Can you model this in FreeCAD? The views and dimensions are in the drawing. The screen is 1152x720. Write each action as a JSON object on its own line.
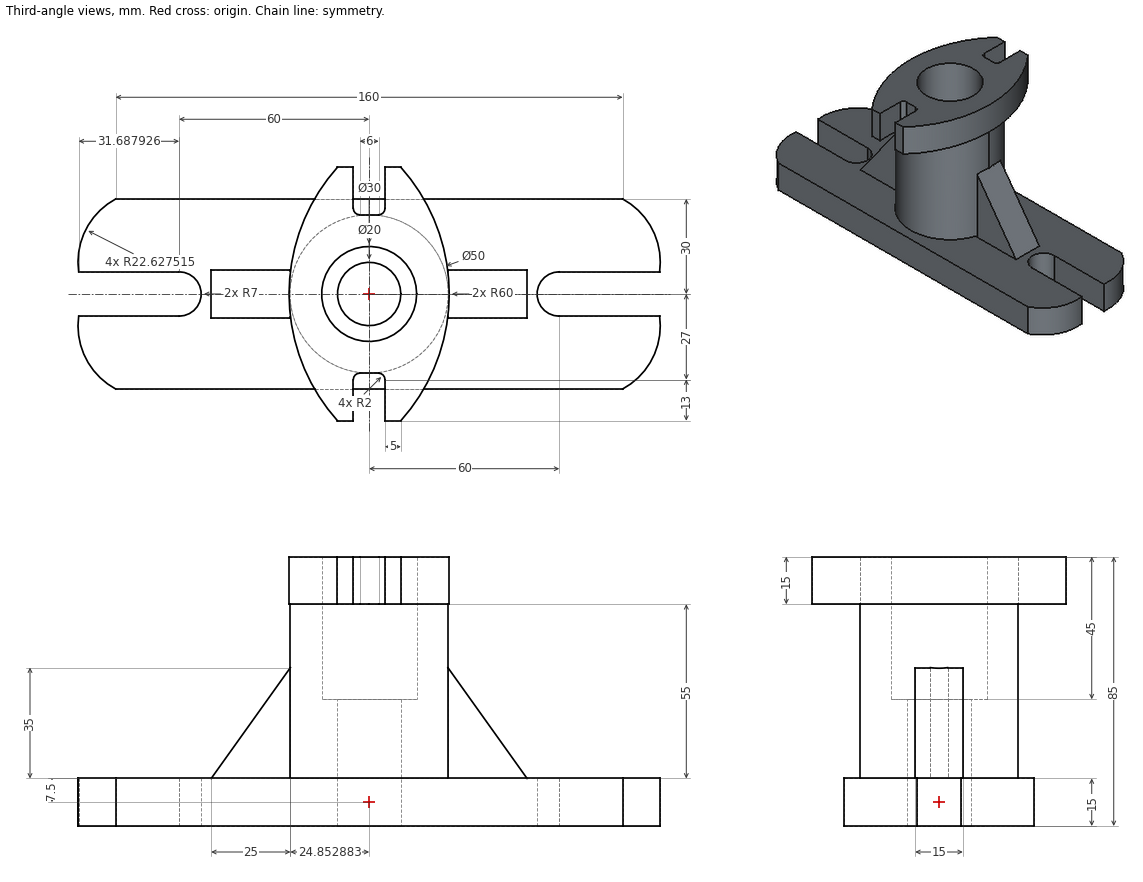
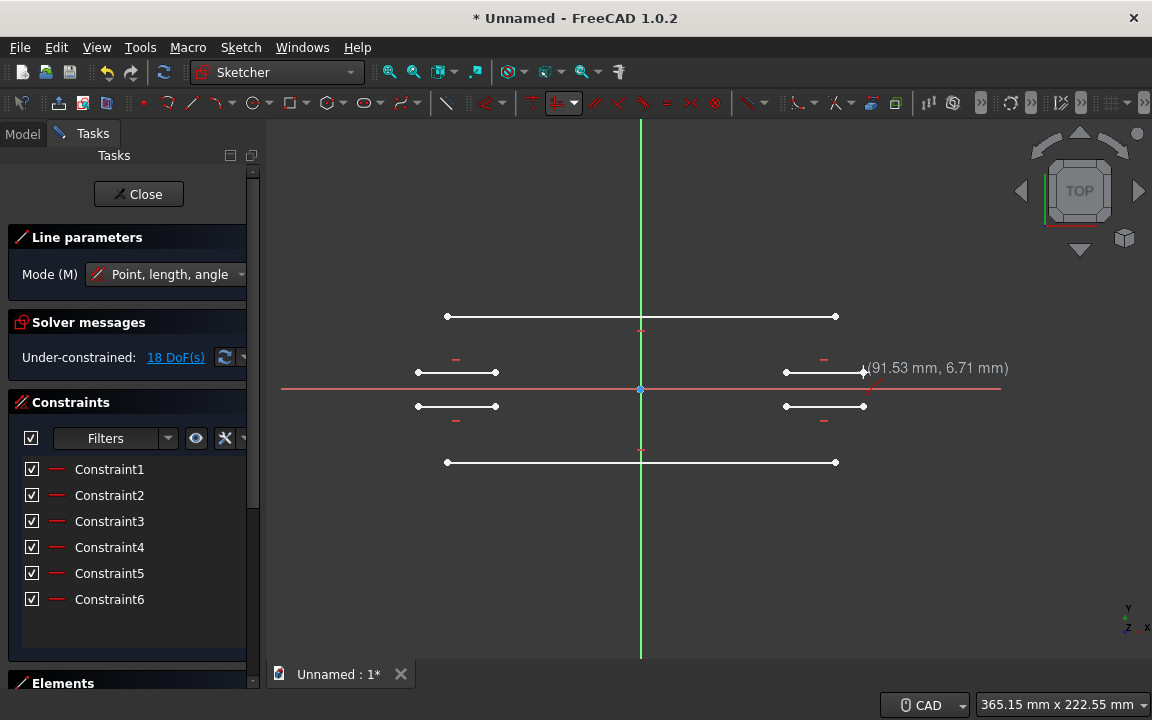
{"action": "key", "text": "g 3 a"}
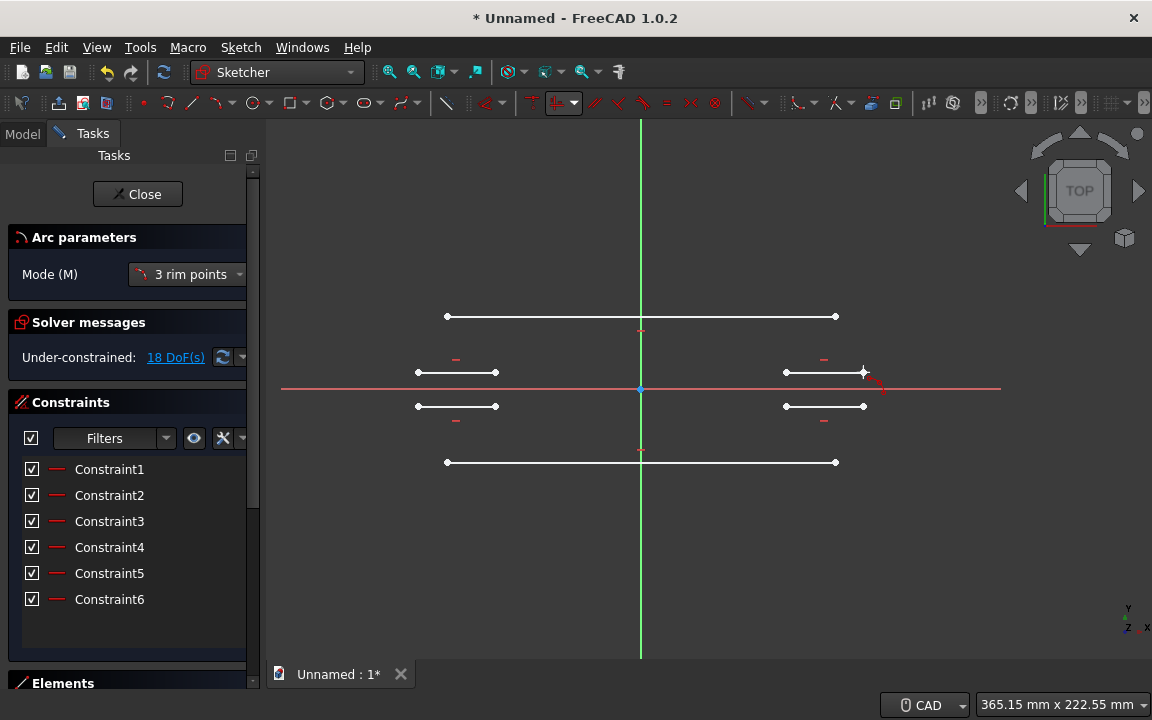
{"action": "left_click", "coordinate": [447, 317]}
{"action": "left_click", "coordinate": [418, 373]}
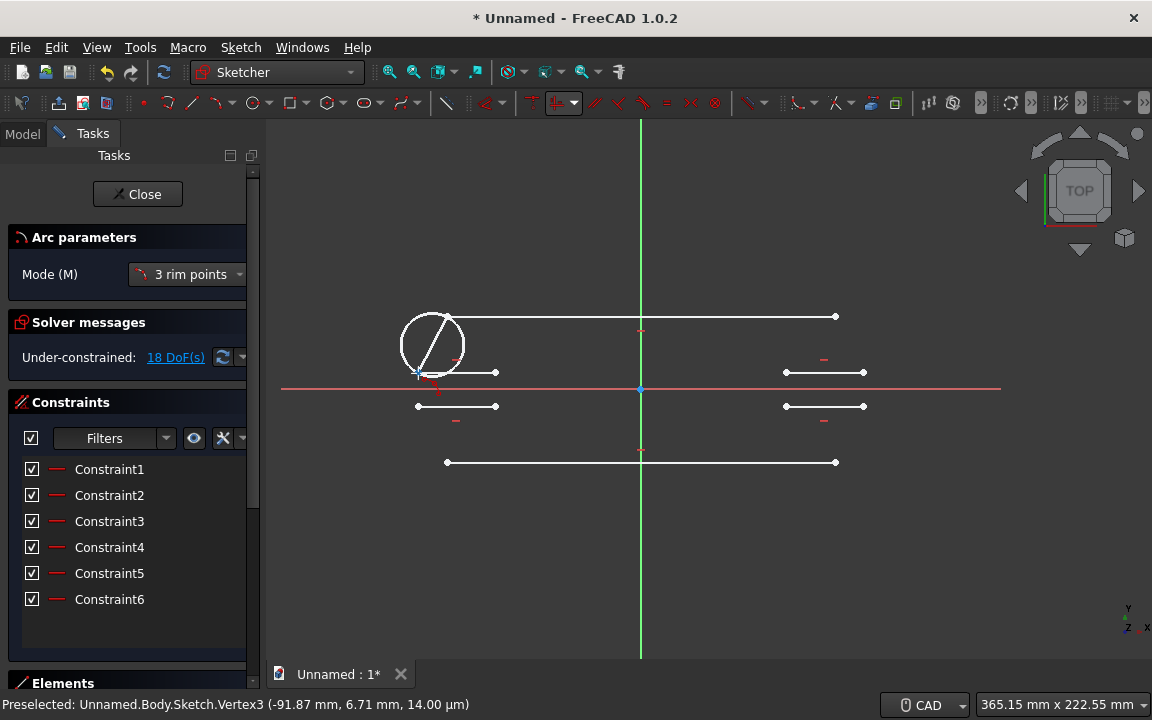
{"action": "scroll", "coordinate": [424, 340], "scroll_direction": "up", "scroll_amount": 3}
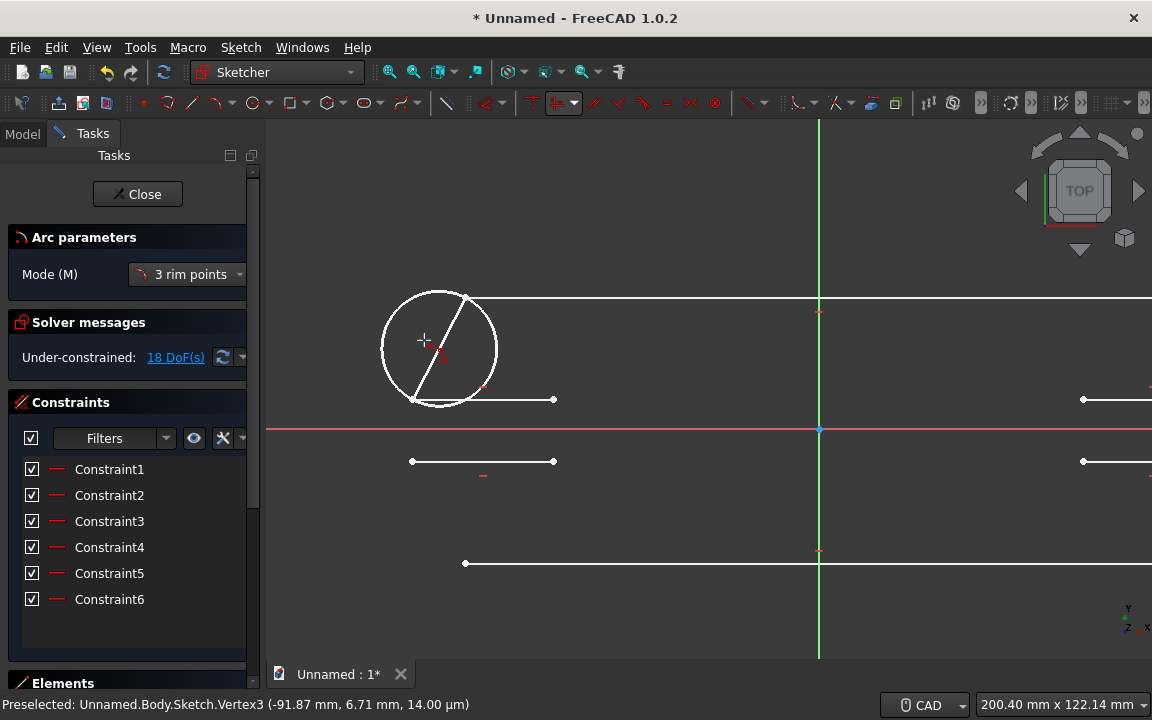
{"action": "left_click", "coordinate": [424, 340]}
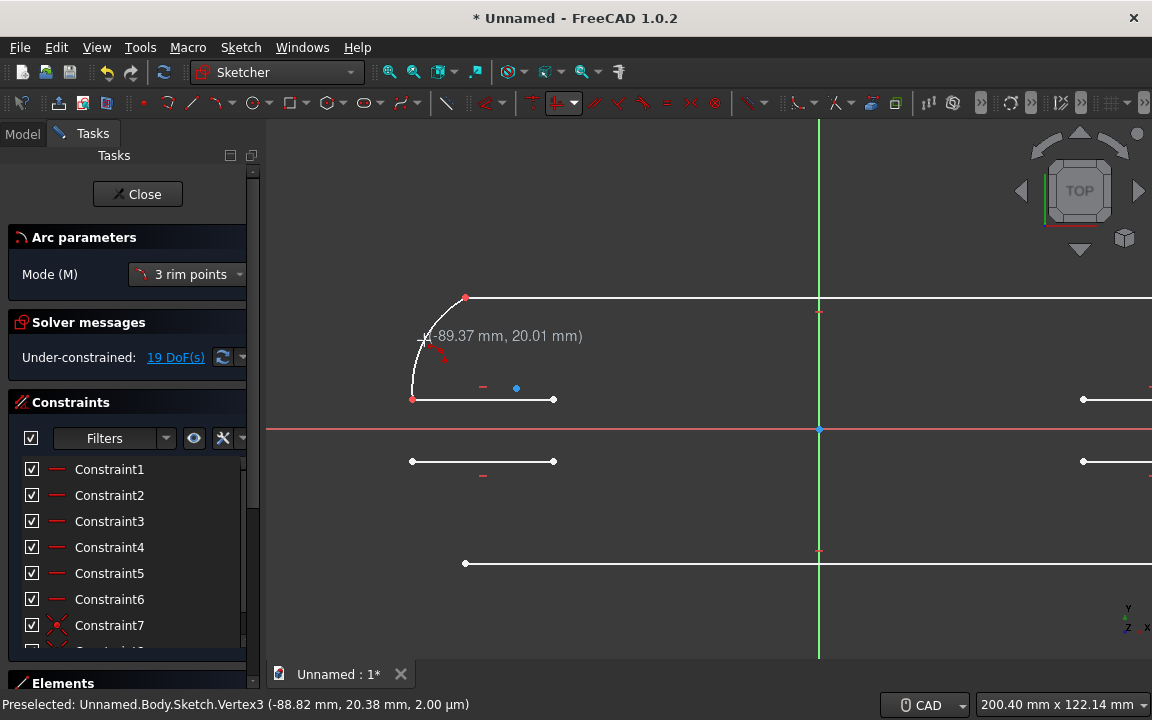
{"action": "left_click", "coordinate": [553, 400]}
{"action": "left_click", "coordinate": [553, 462]}
{"action": "left_click", "coordinate": [579, 448]}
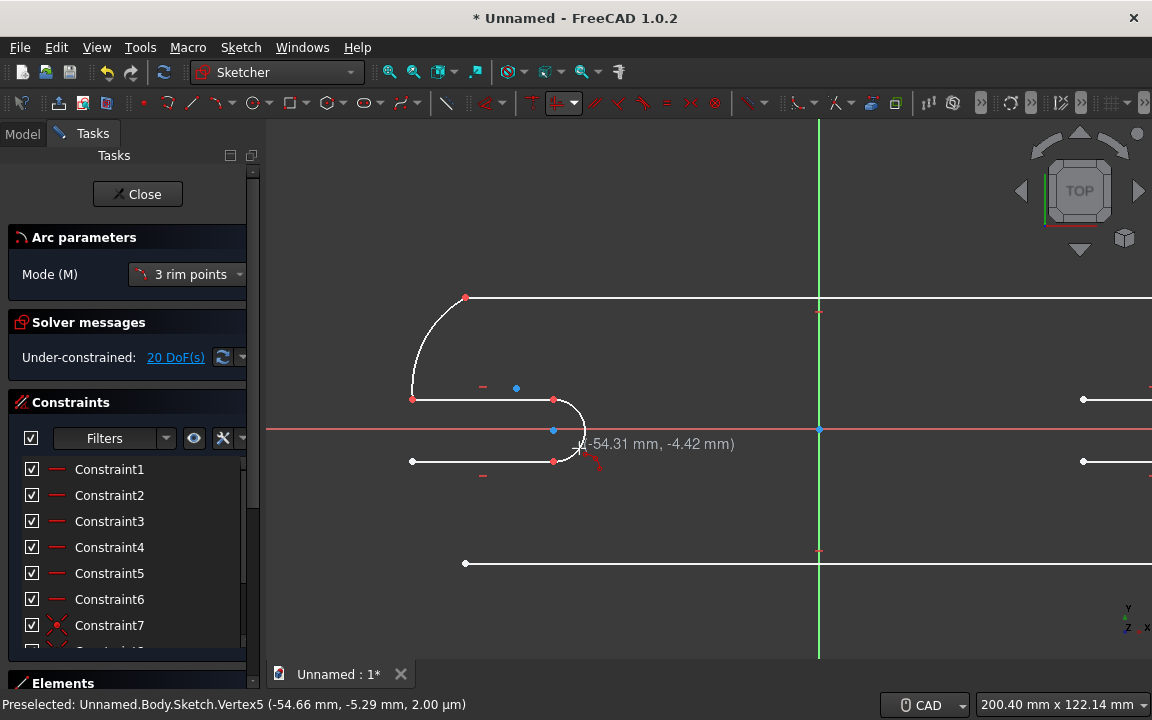
{"action": "left_click", "coordinate": [413, 462]}
{"action": "left_click", "coordinate": [466, 564]}
{"action": "left_click", "coordinate": [424, 519]}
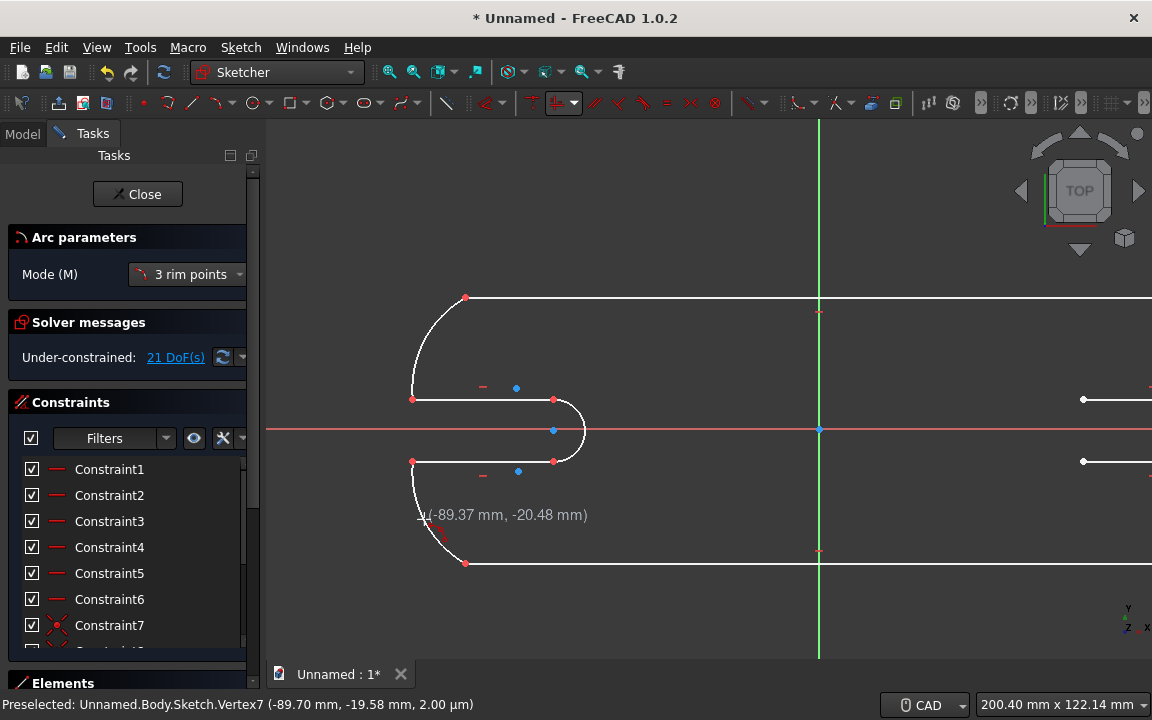
{"action": "scroll", "coordinate": [423, 340], "scroll_direction": "down", "scroll_amount": 3}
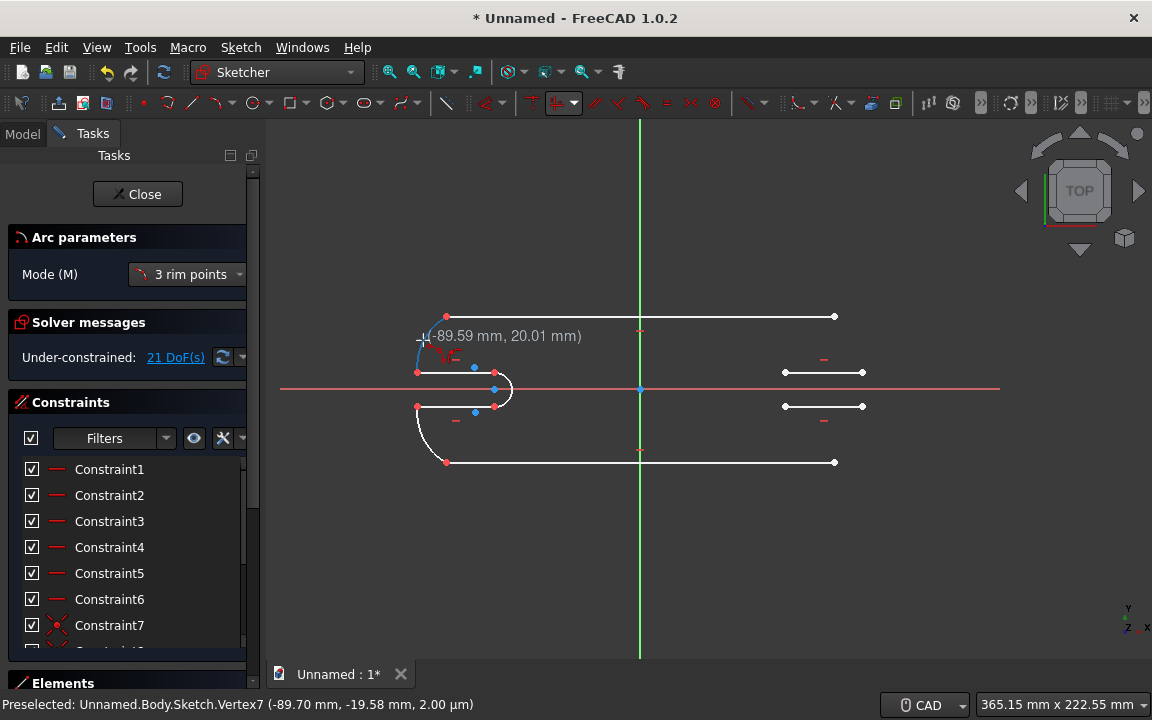
{"action": "left_click", "coordinate": [835, 463]}
{"action": "left_click", "coordinate": [863, 407]}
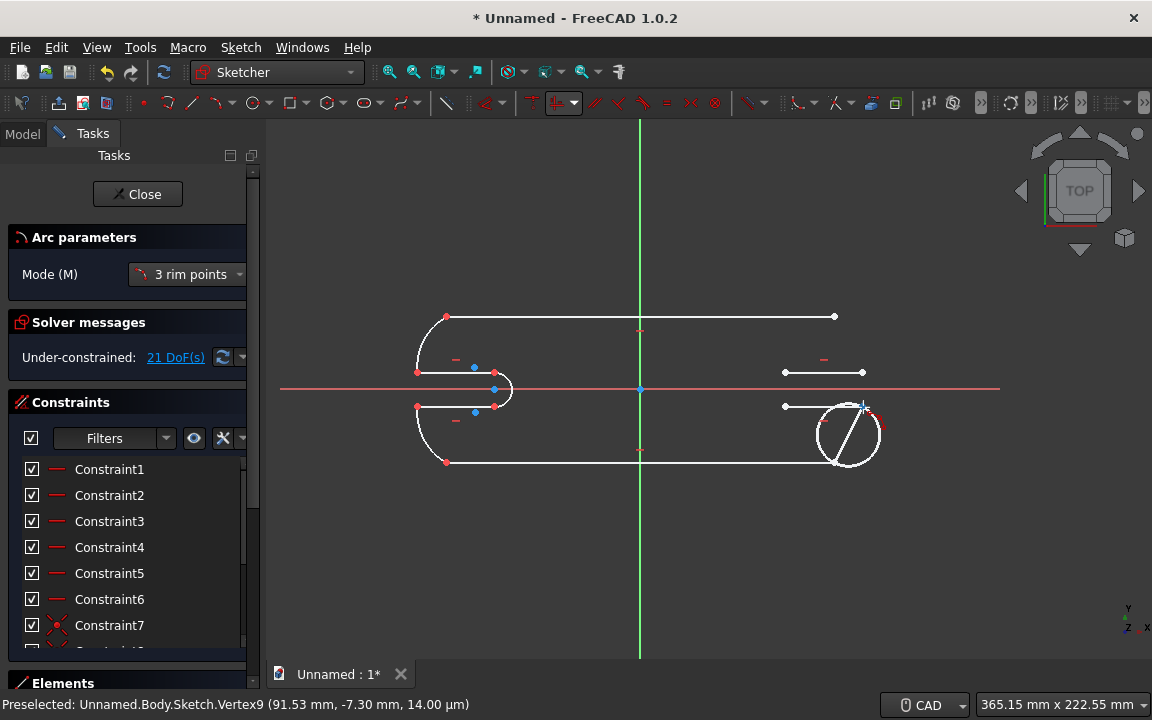
{"action": "scroll", "coordinate": [857, 439], "scroll_direction": "up", "scroll_amount": 3}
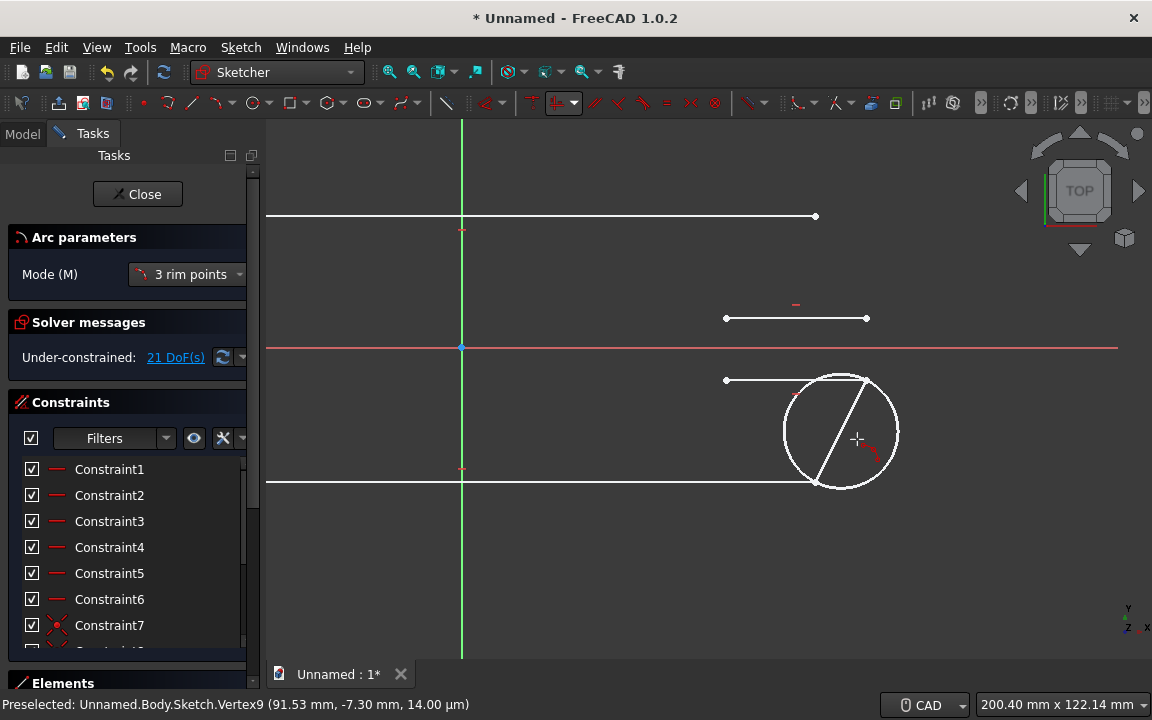
{"action": "left_click", "coordinate": [857, 438]}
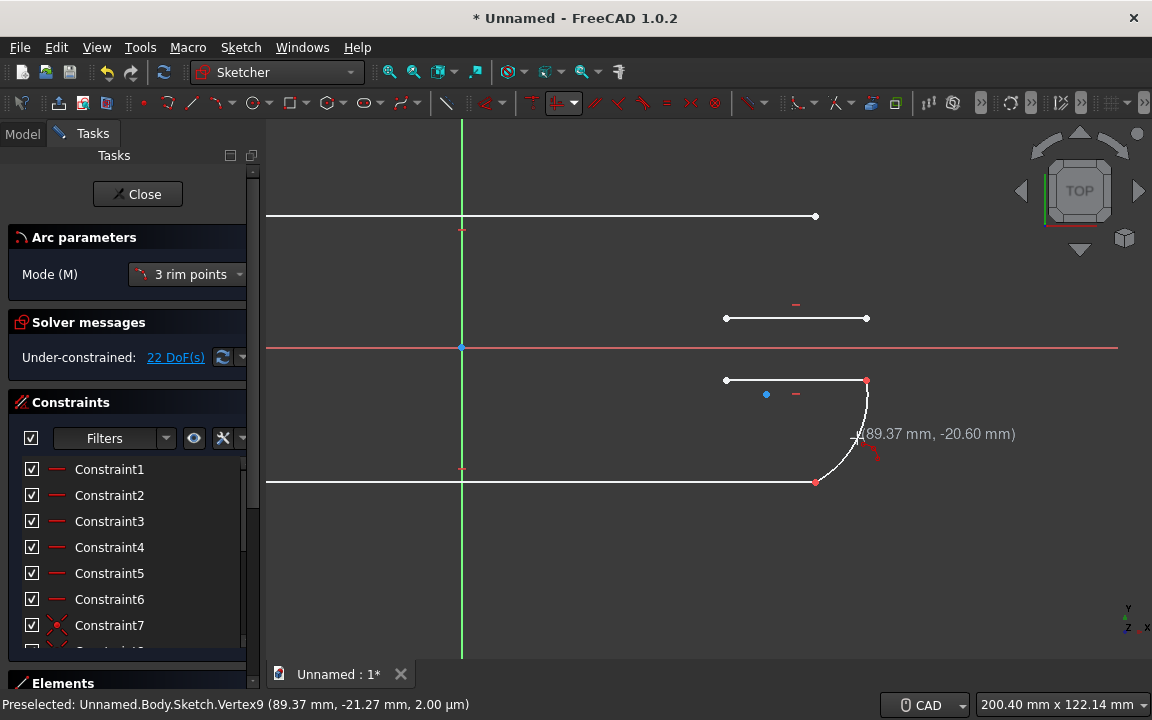
{"action": "left_click", "coordinate": [726, 380]}
{"action": "left_click", "coordinate": [726, 318]}
{"action": "left_click", "coordinate": [702, 330]}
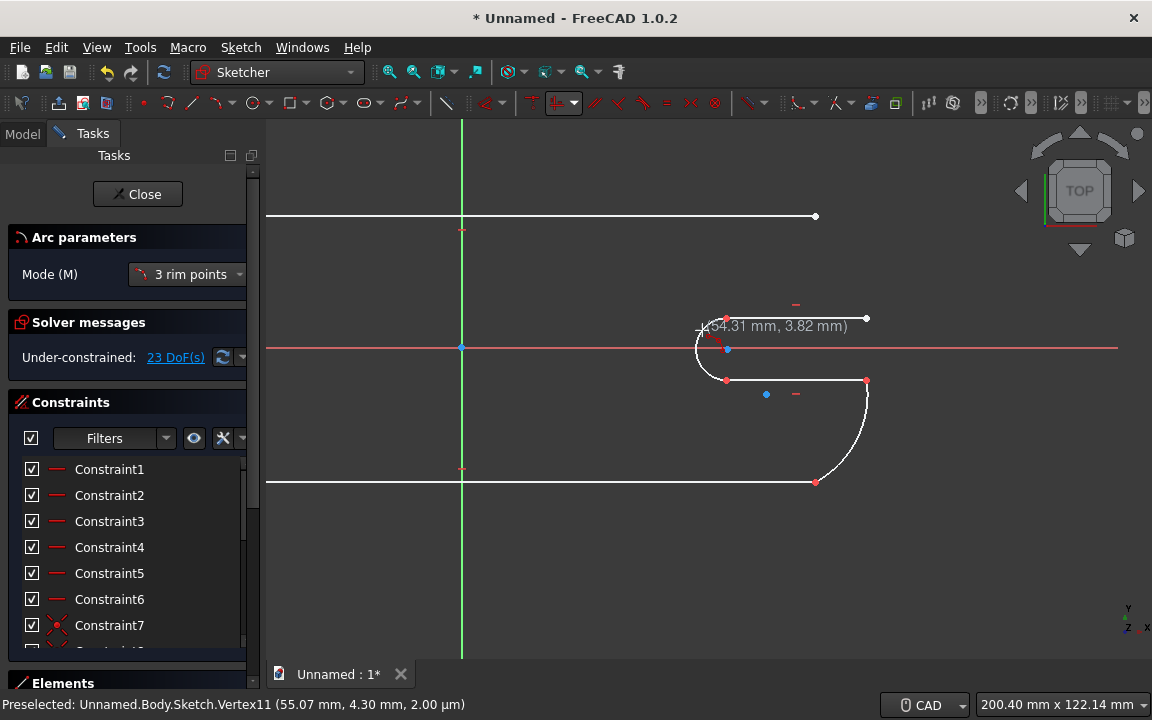
{"action": "left_click", "coordinate": [867, 318]}
{"action": "left_click", "coordinate": [816, 216]}
{"action": "left_click", "coordinate": [857, 258]}
{"action": "key", "text": "Escape"}